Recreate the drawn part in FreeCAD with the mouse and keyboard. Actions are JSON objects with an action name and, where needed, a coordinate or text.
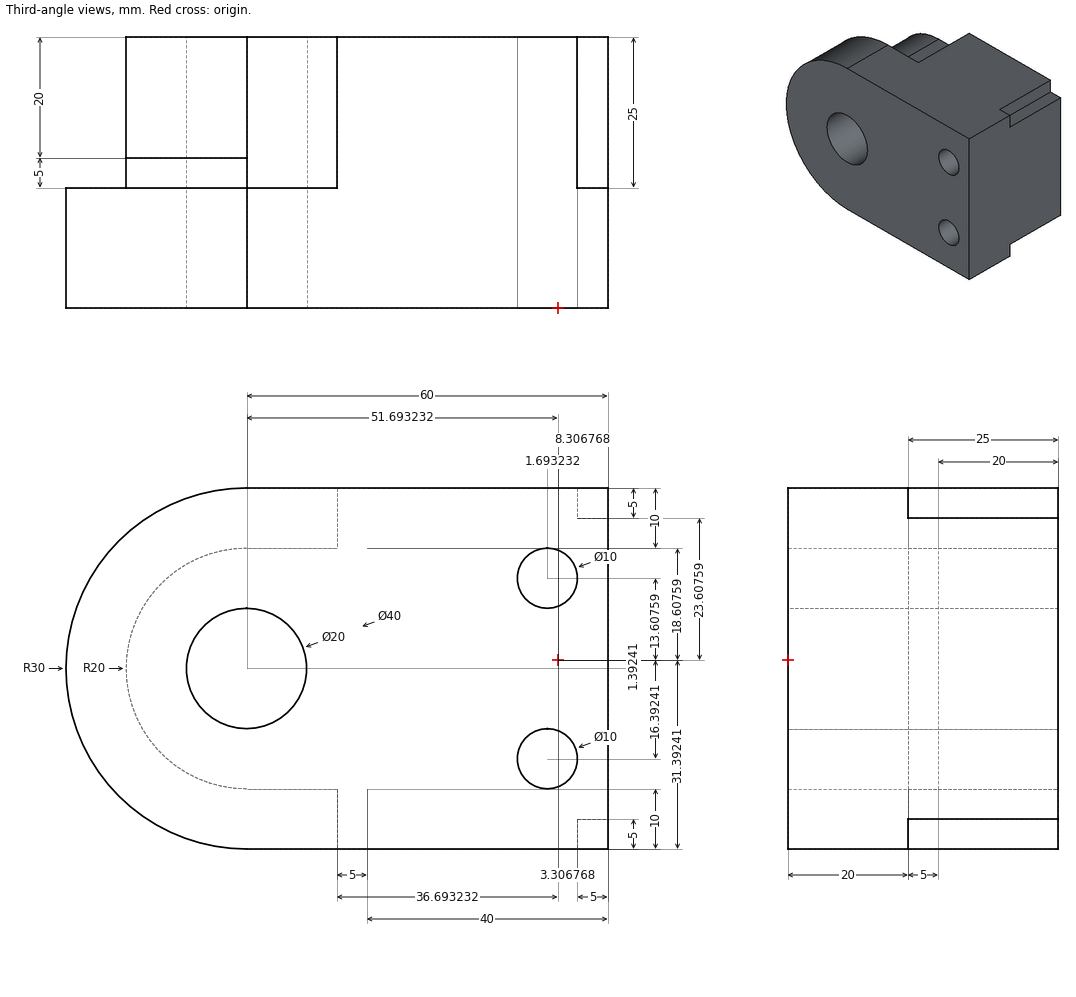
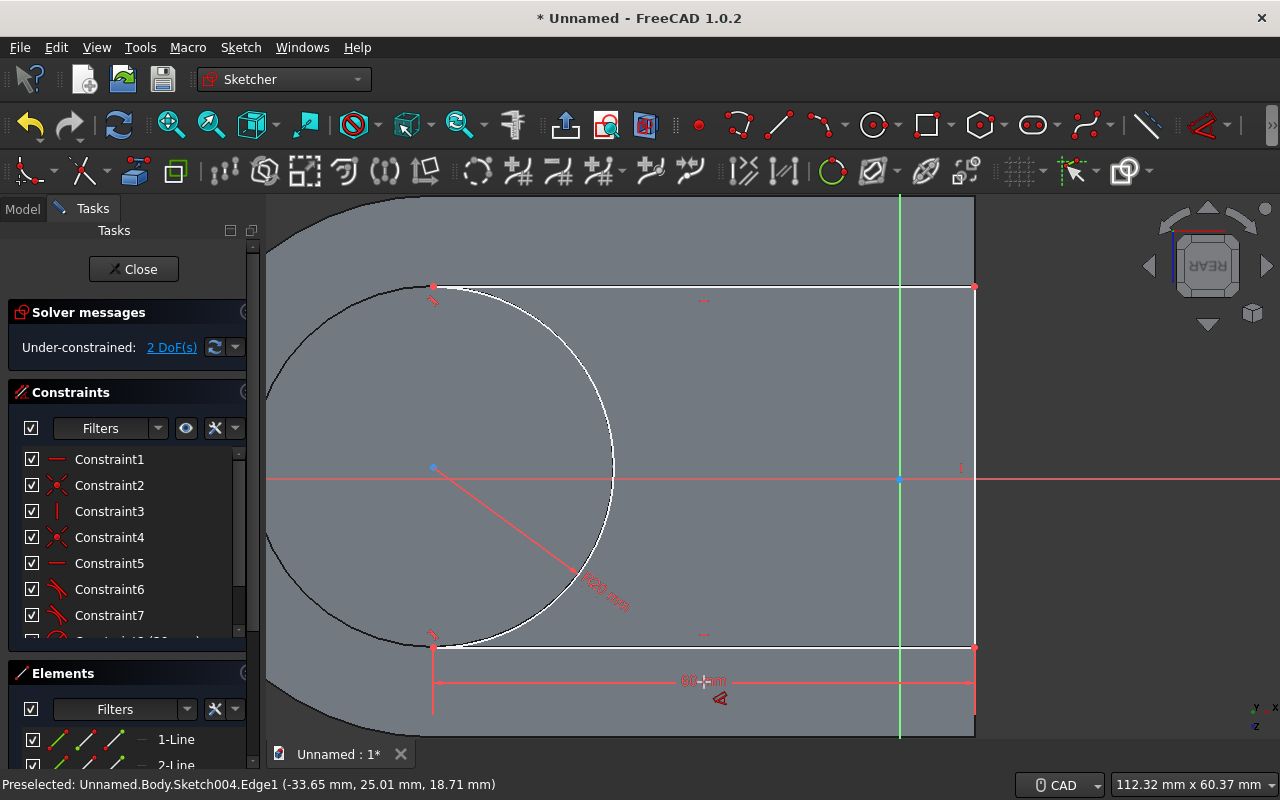
{"action": "scroll", "coordinate": [433, 467], "scroll_direction": "up", "scroll_amount": 6}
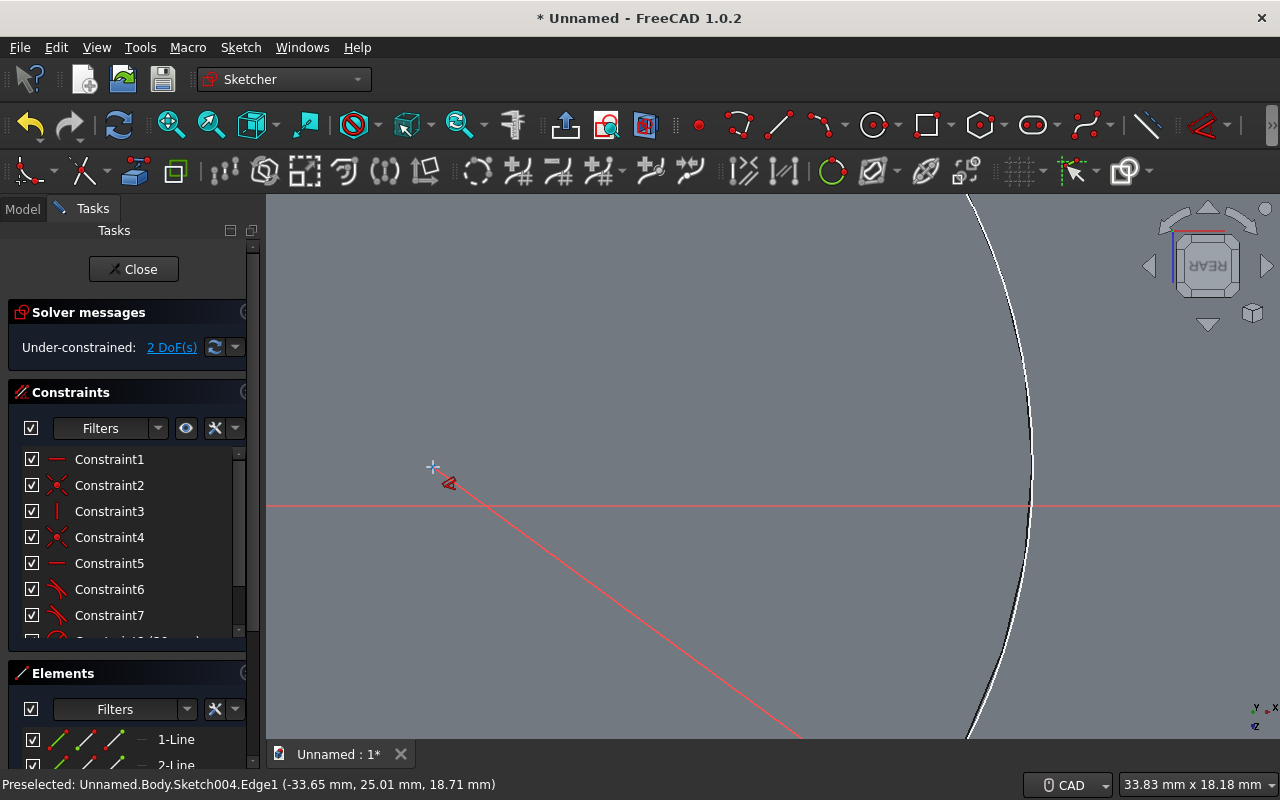
{"action": "left_click", "coordinate": [433, 467]}
{"action": "left_click", "coordinate": [399, 487]}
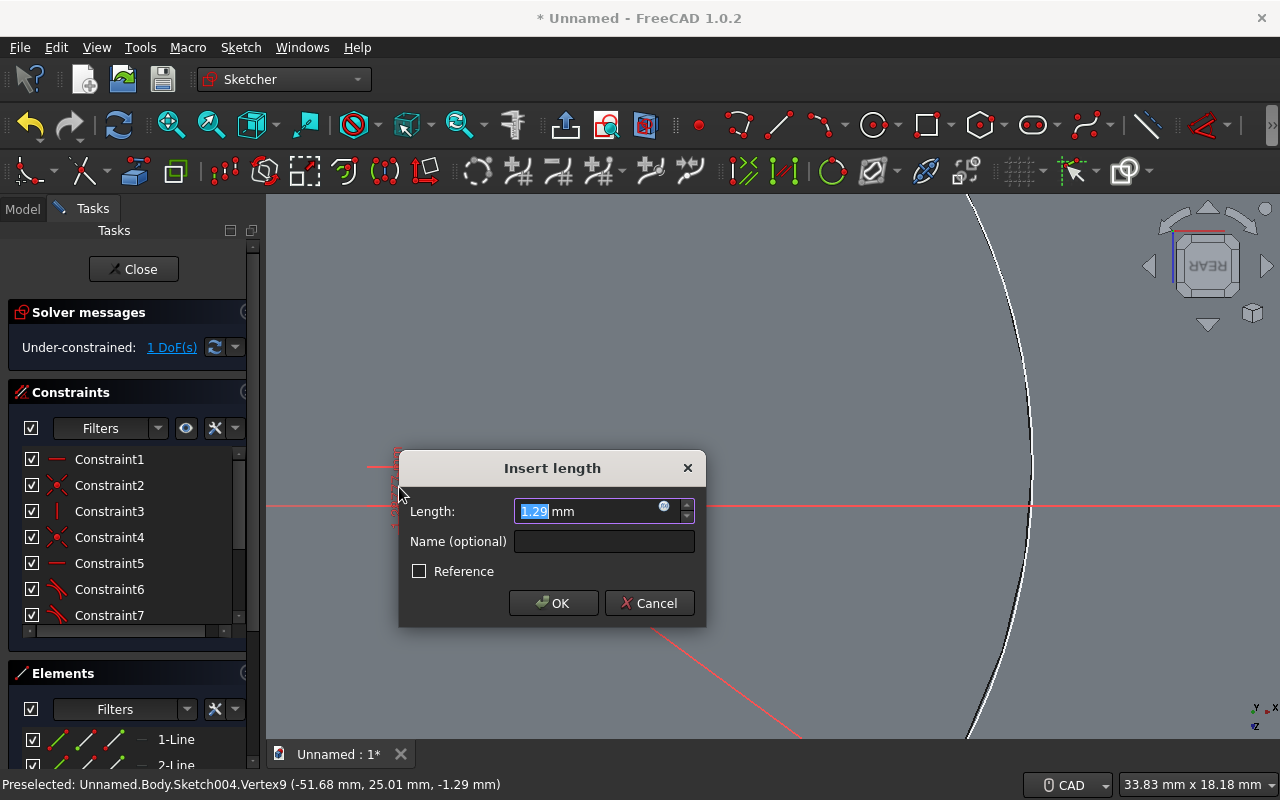
{"action": "type", "text": "1.39241"}
{"action": "key", "text": "Return"}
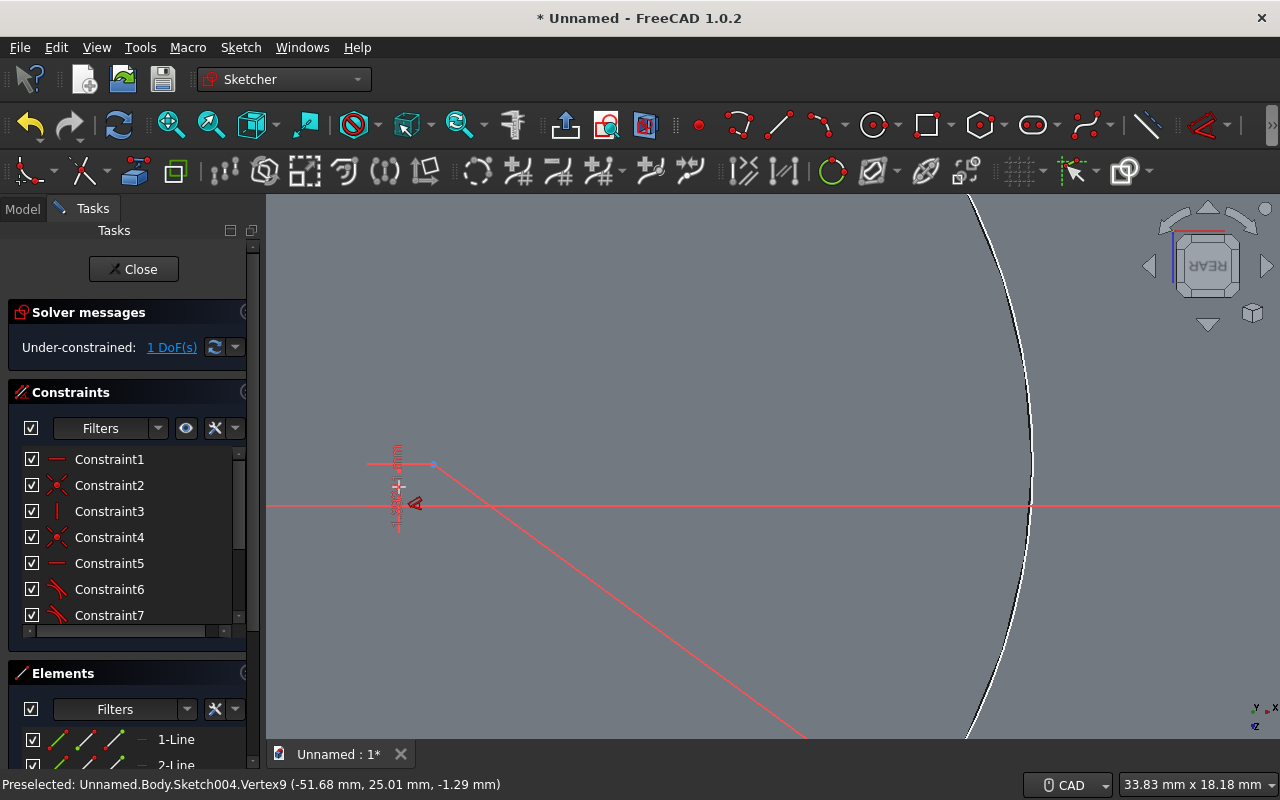
{"action": "scroll", "coordinate": [434, 468], "scroll_direction": "down", "scroll_amount": 6}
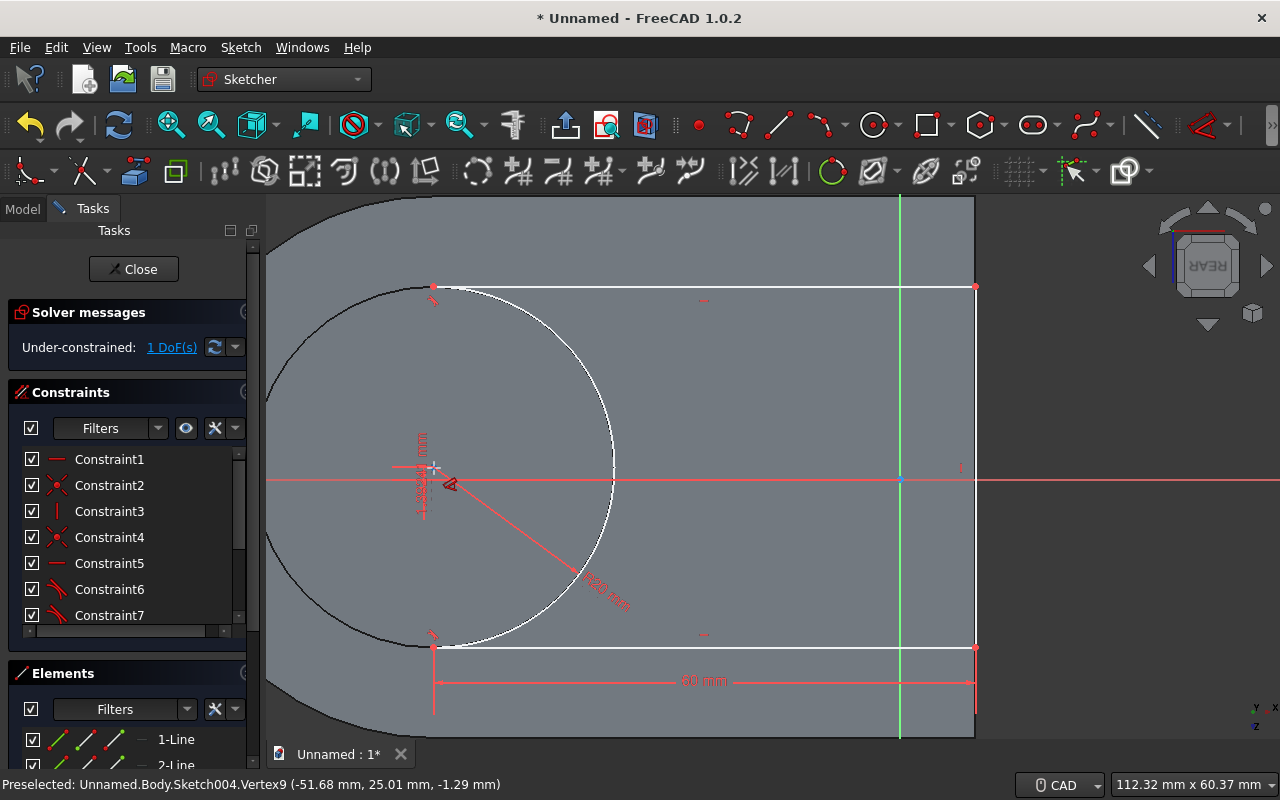
{"action": "left_click", "coordinate": [976, 648]}
{"action": "left_click", "coordinate": [938, 682]}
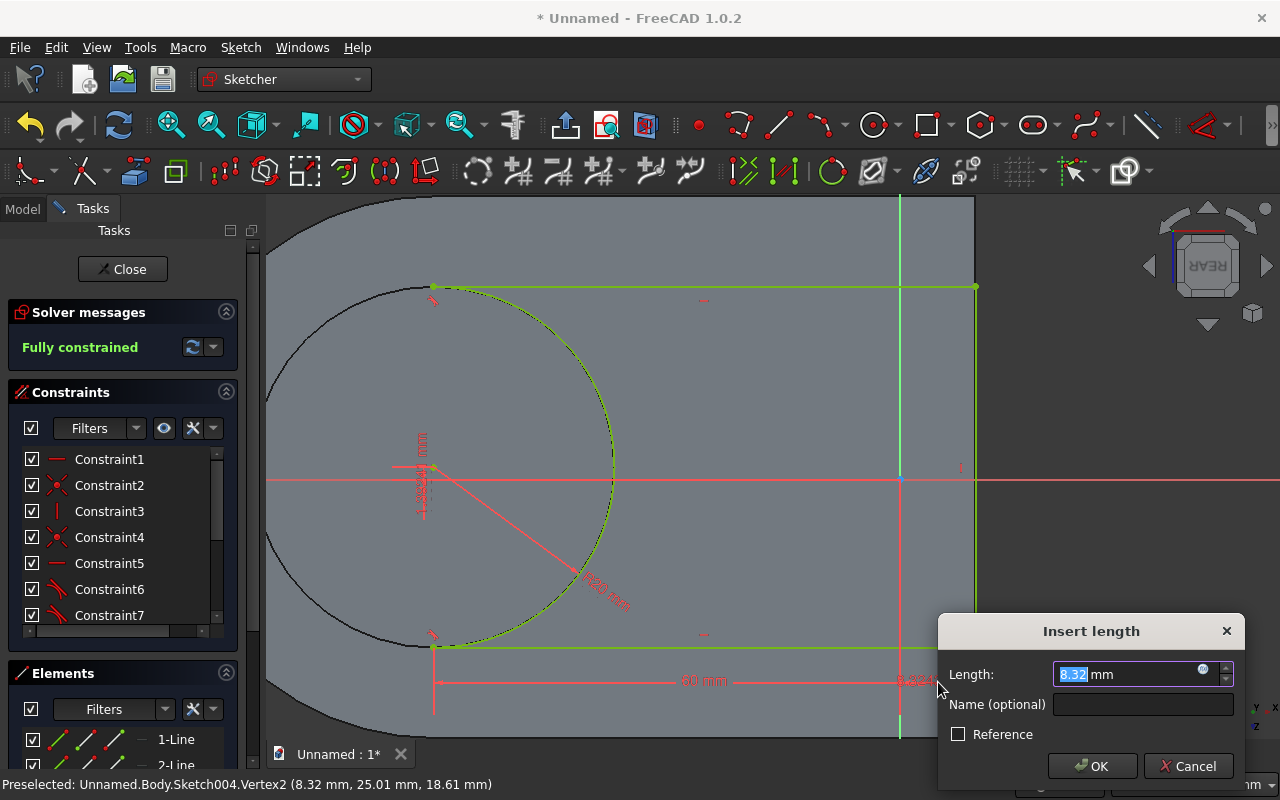
{"action": "type", "text": "8.306768"}
{"action": "key", "text": "Return"}
{"action": "key", "text": "Escape"}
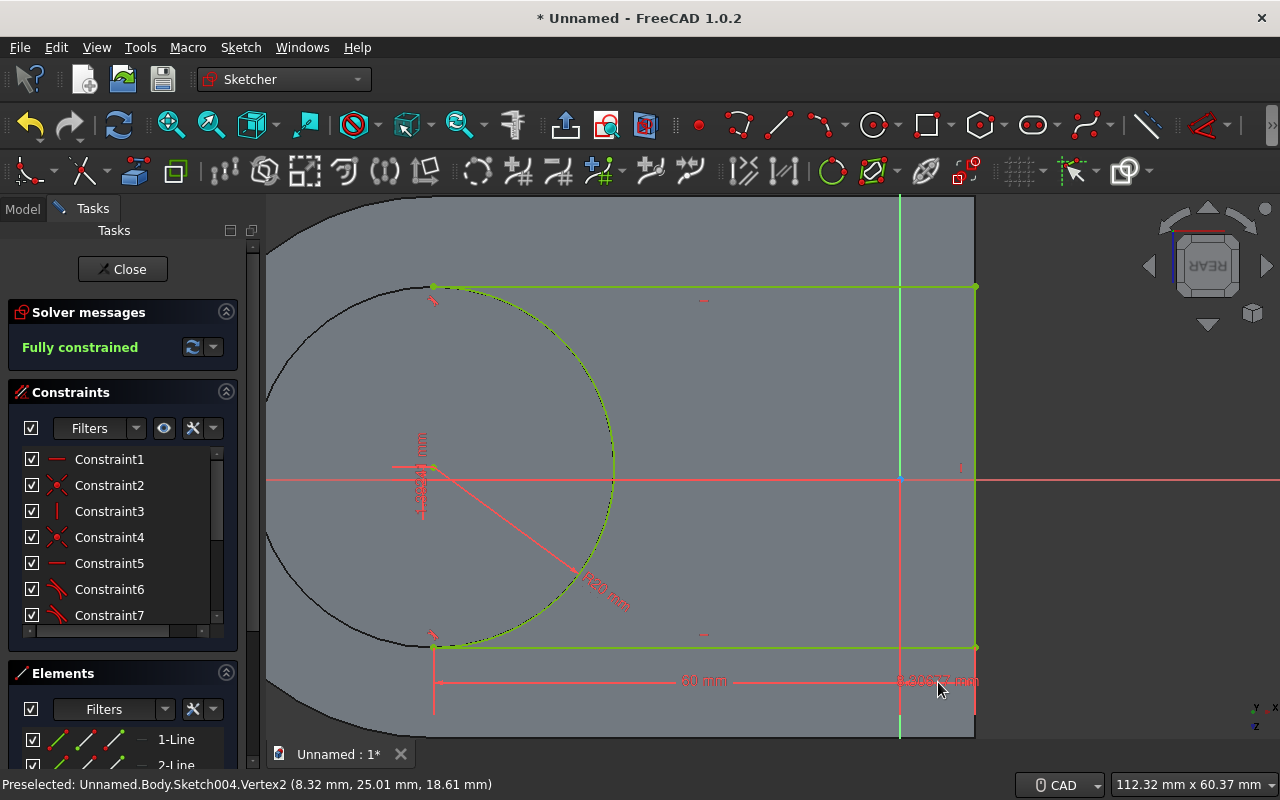
{"action": "left_click", "coordinate": [123, 269]}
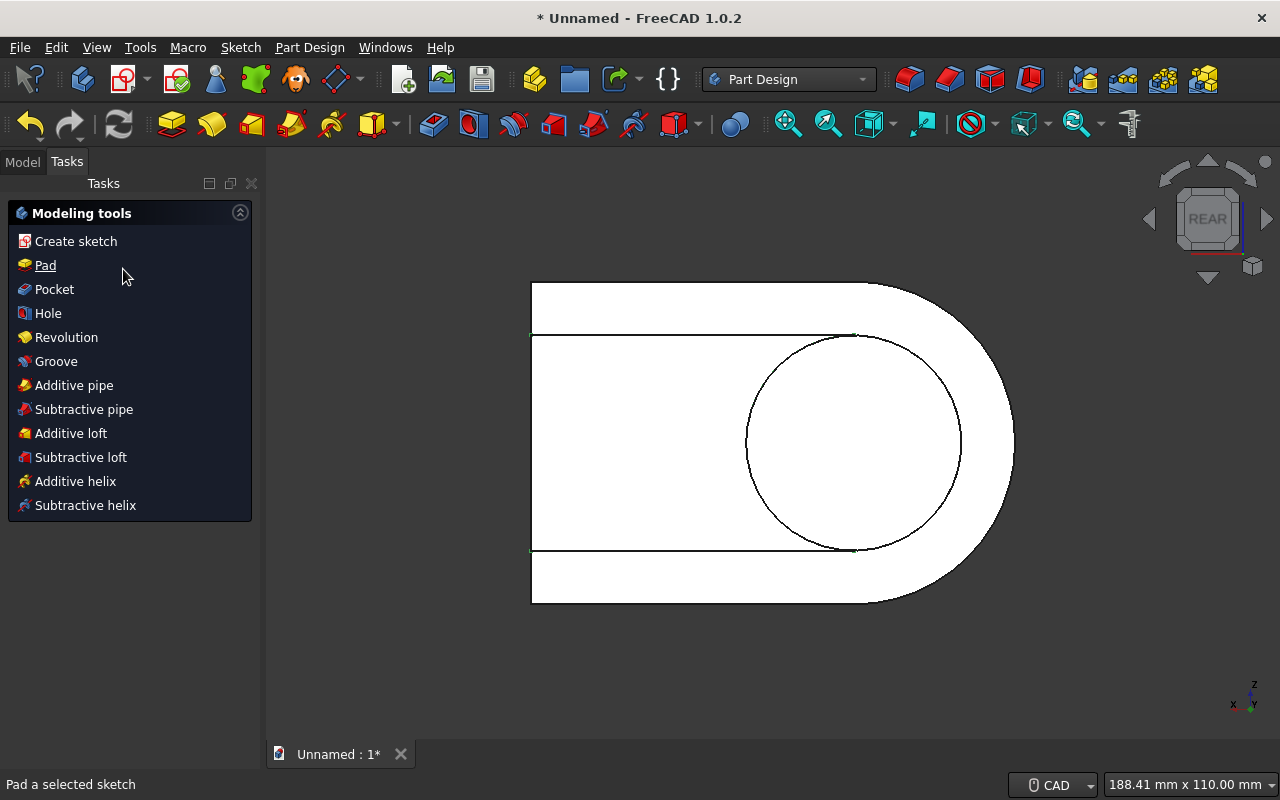
{"action": "left_click", "coordinate": [172, 124]}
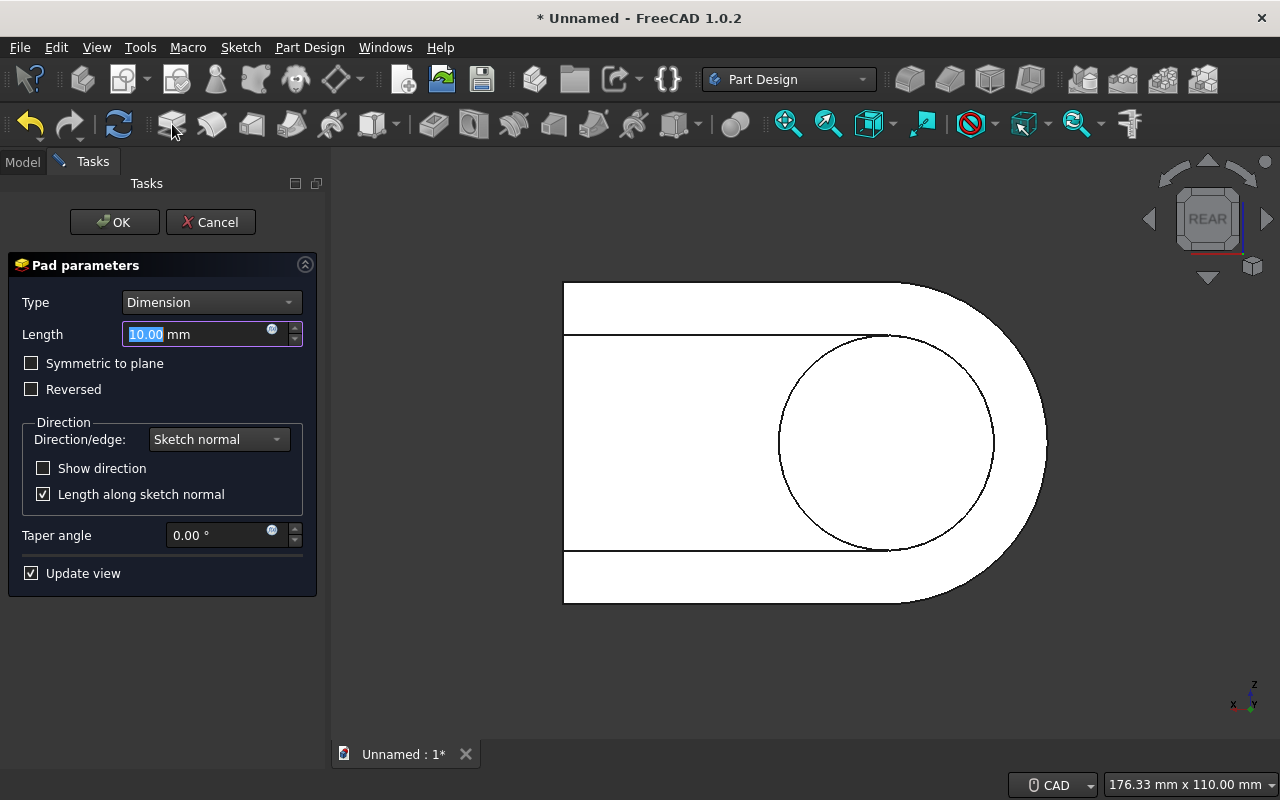
{"action": "type", "text": "20"}
{"action": "key", "text": "Tab"}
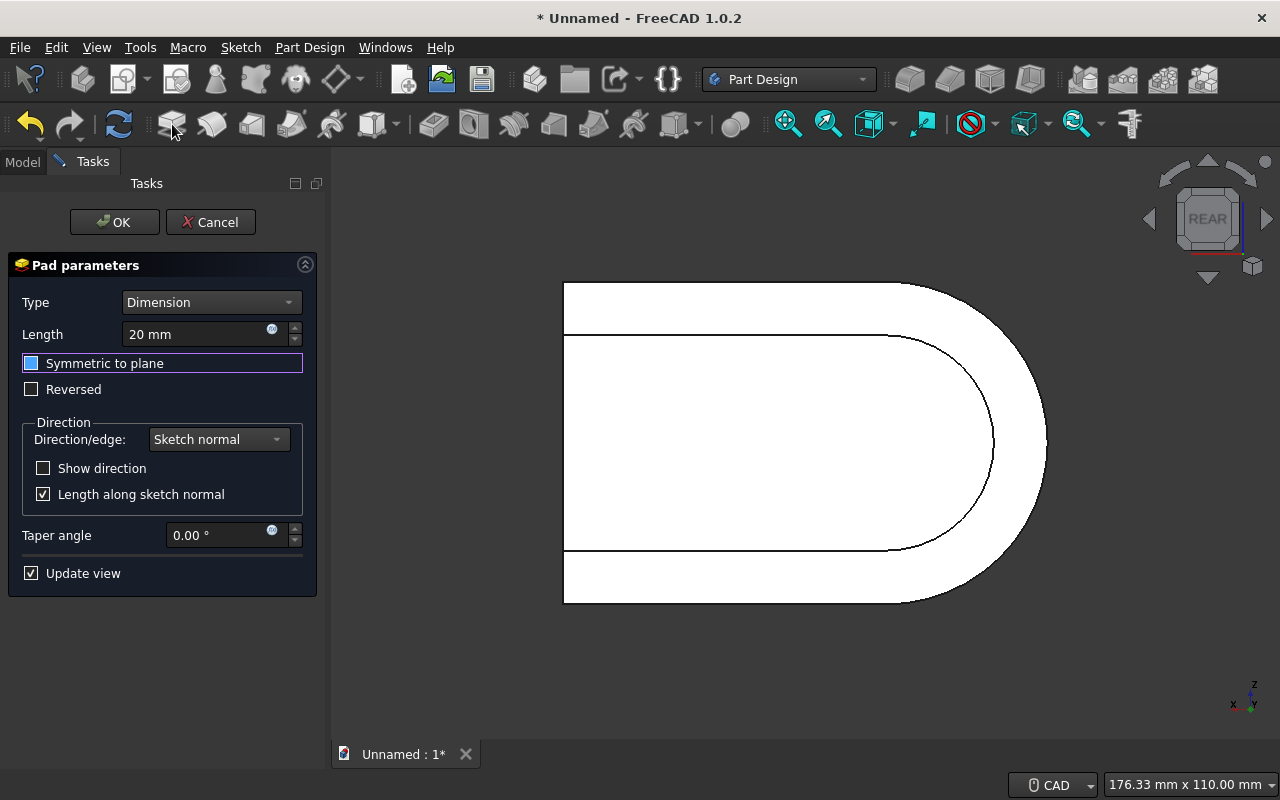
{"action": "left_click", "coordinate": [115, 222]}